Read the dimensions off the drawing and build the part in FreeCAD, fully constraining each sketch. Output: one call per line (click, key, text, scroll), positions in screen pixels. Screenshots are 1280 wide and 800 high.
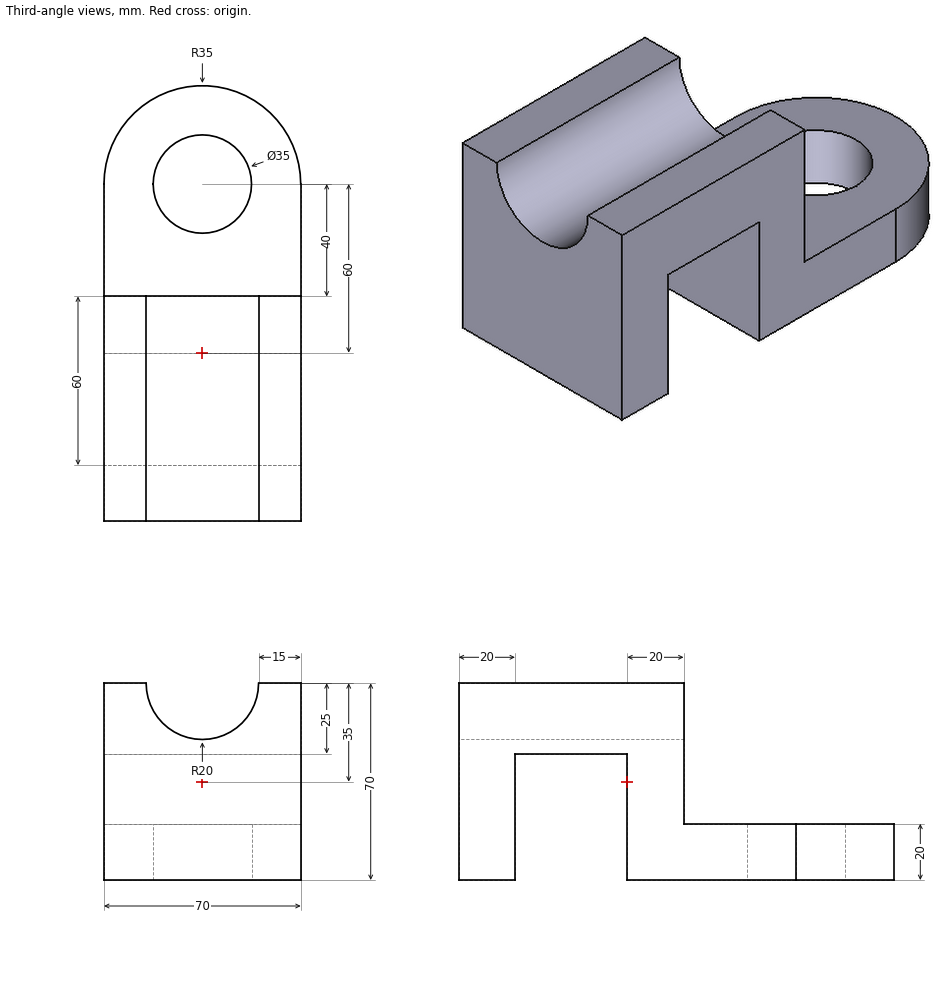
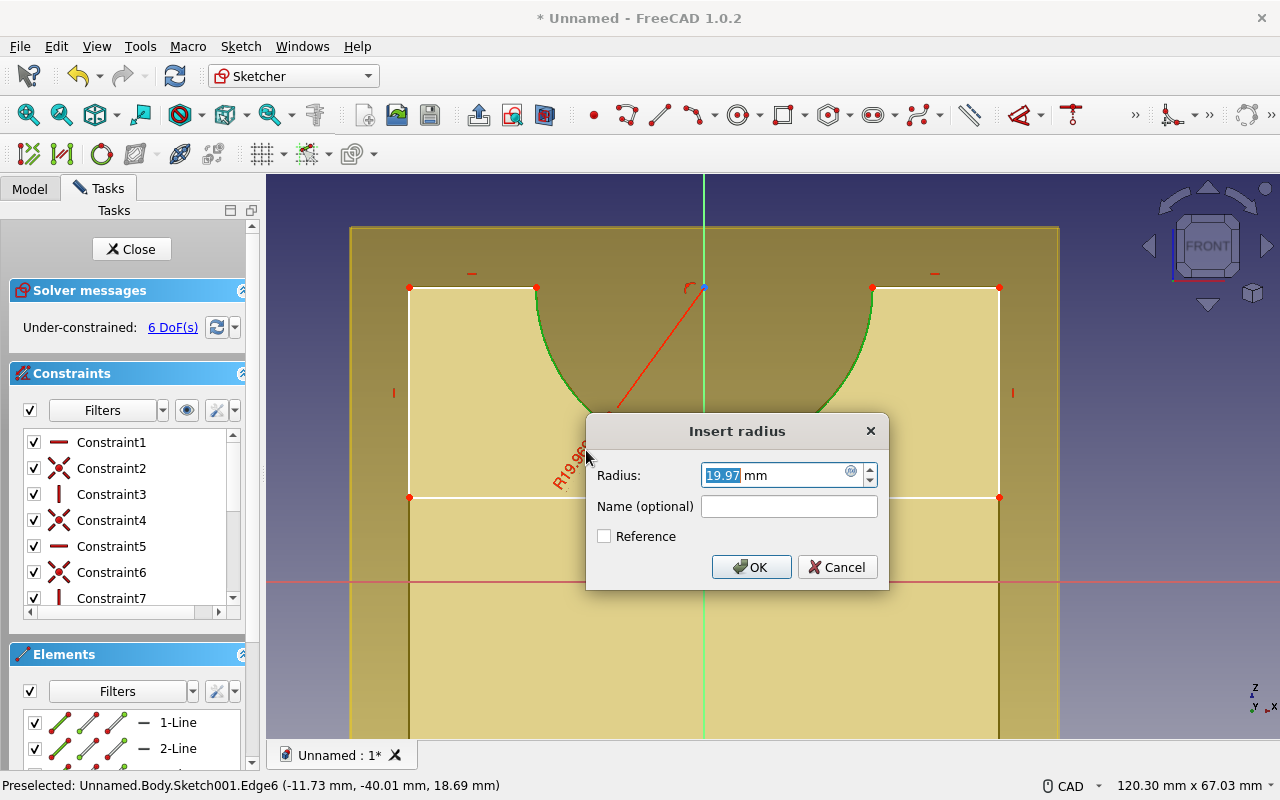
text(20)
key(Return)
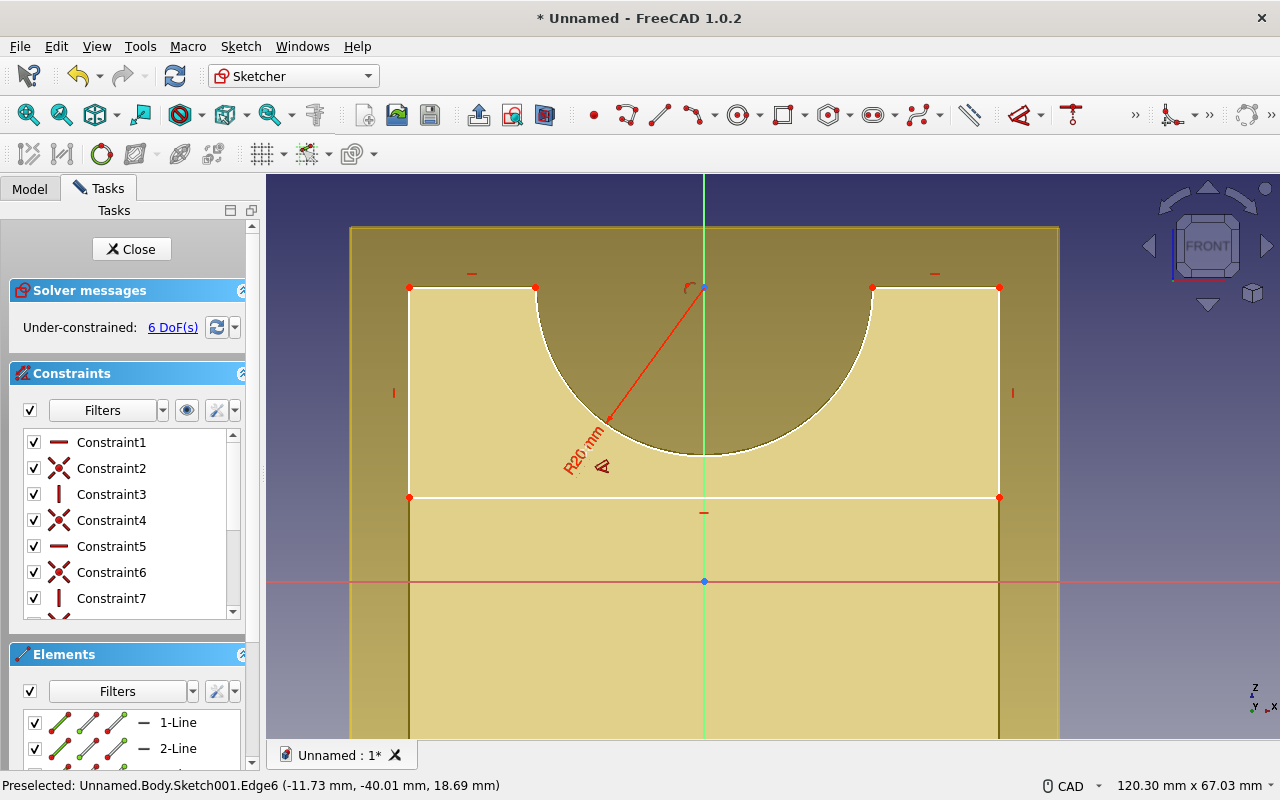
click(911, 288)
click(936, 254)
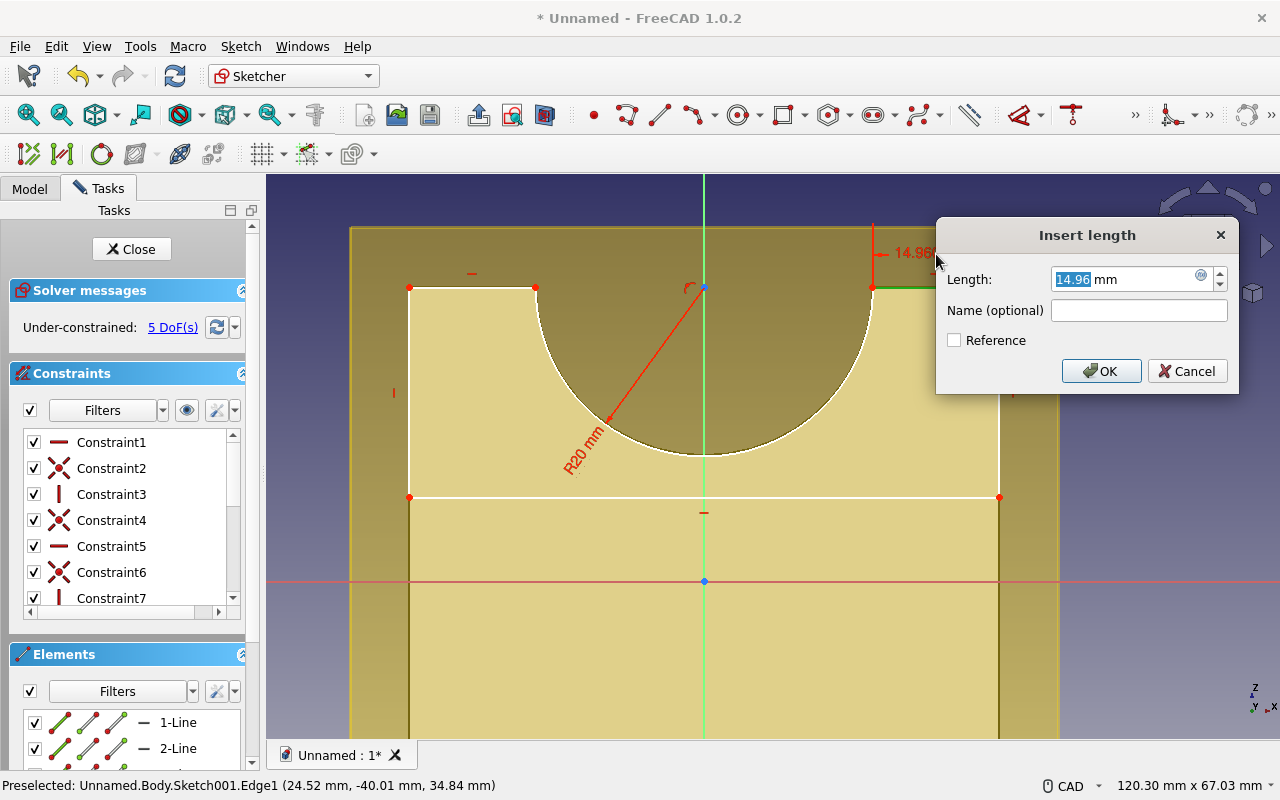
text(15)
key(Return)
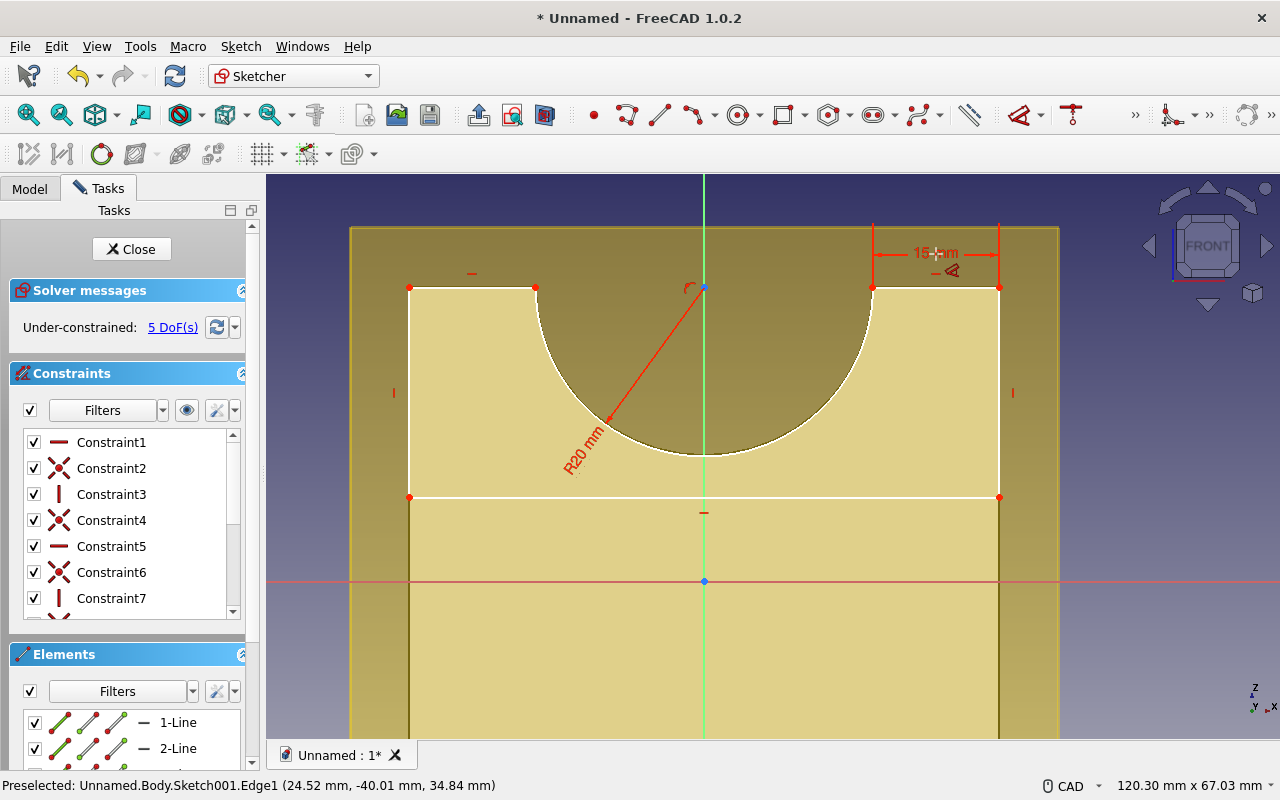
click(999, 351)
click(1033, 393)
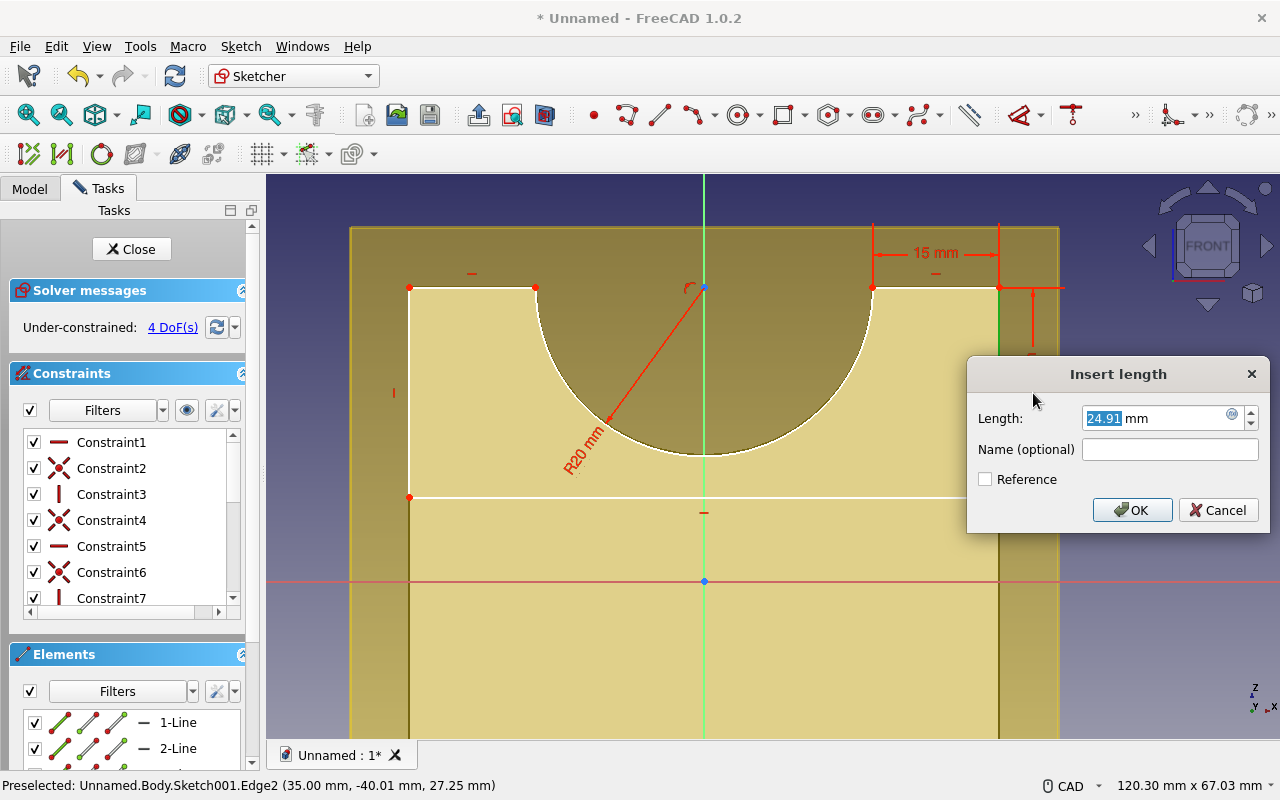
text(25)
key(Return)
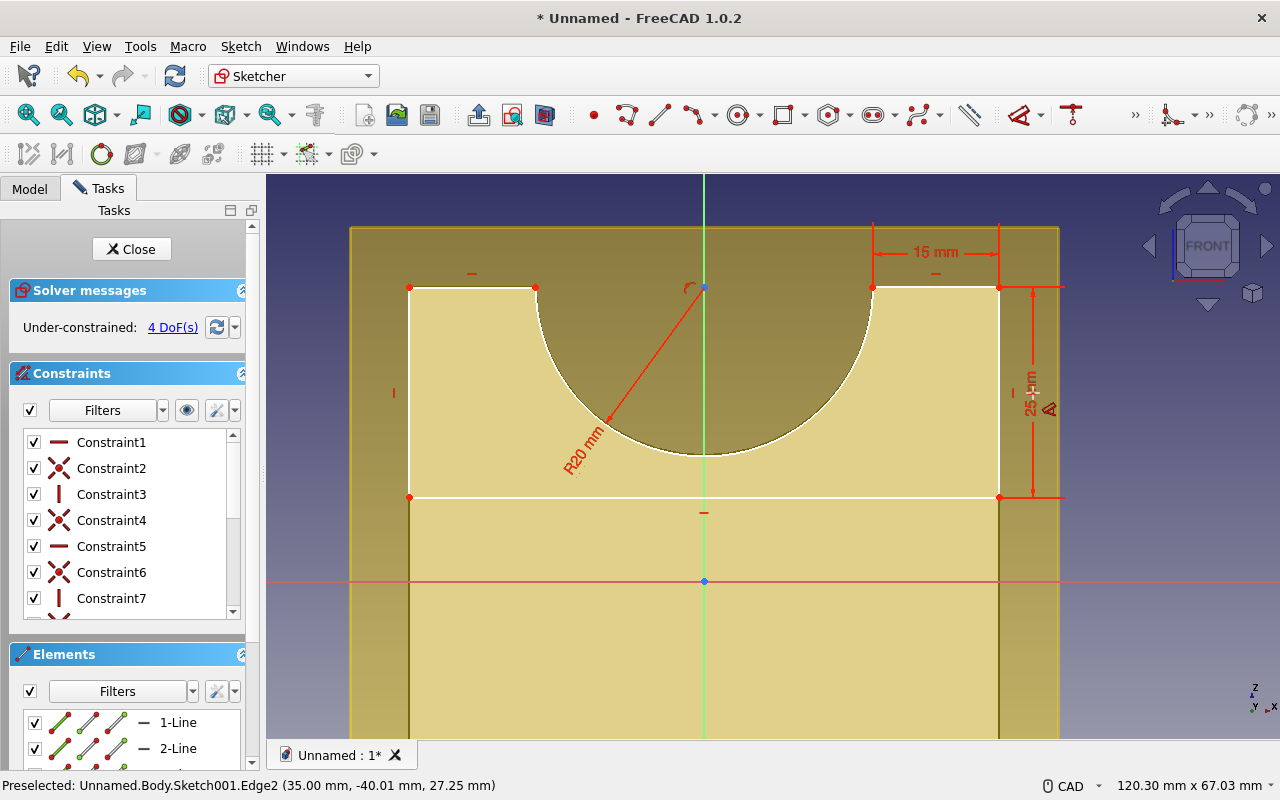
click(822, 498)
click(568, 532)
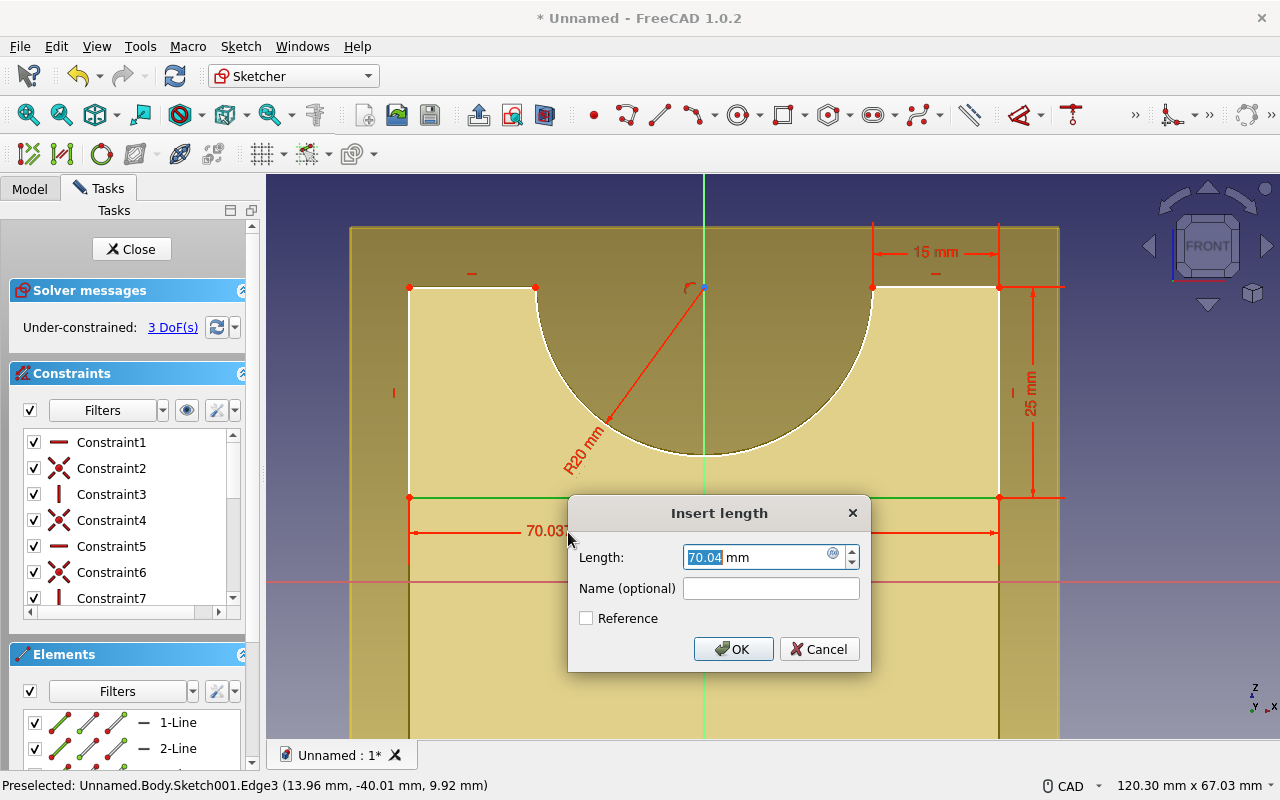
text(70)
key(Return)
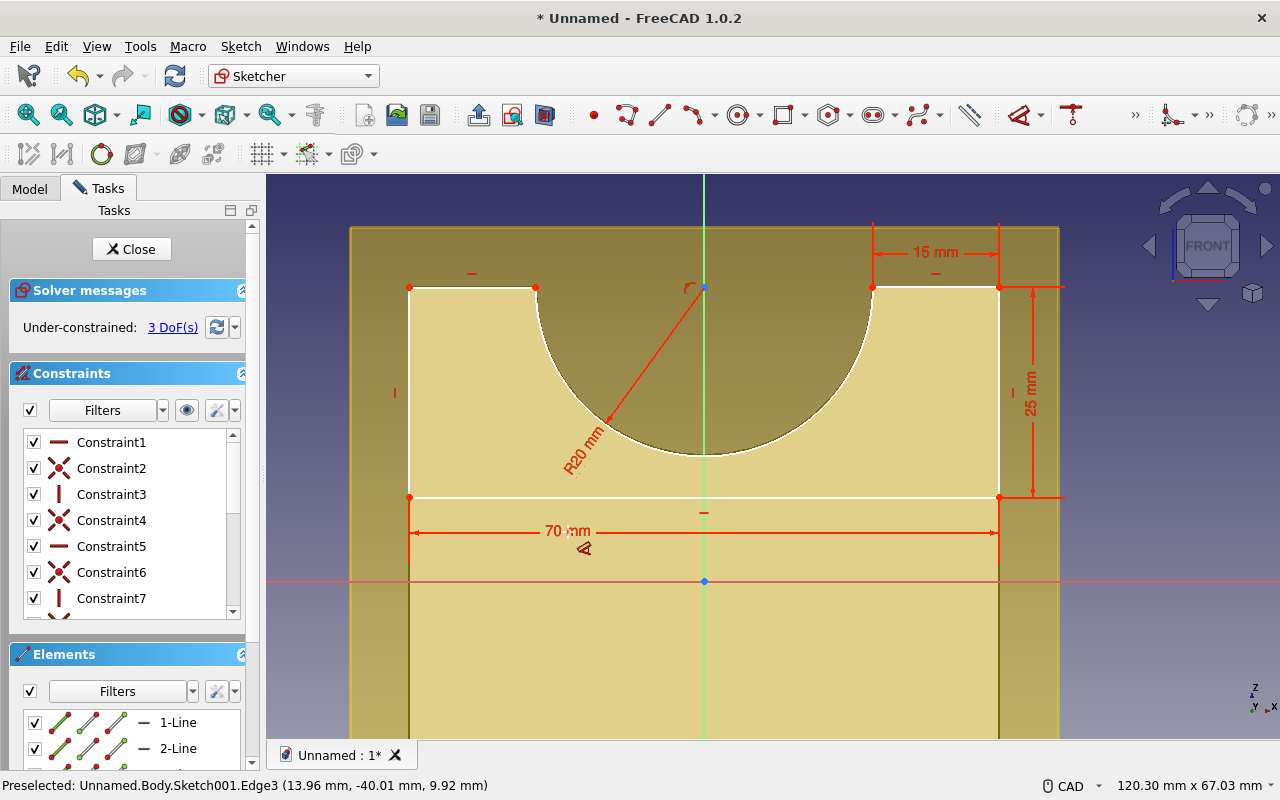
click(409, 435)
click(375, 393)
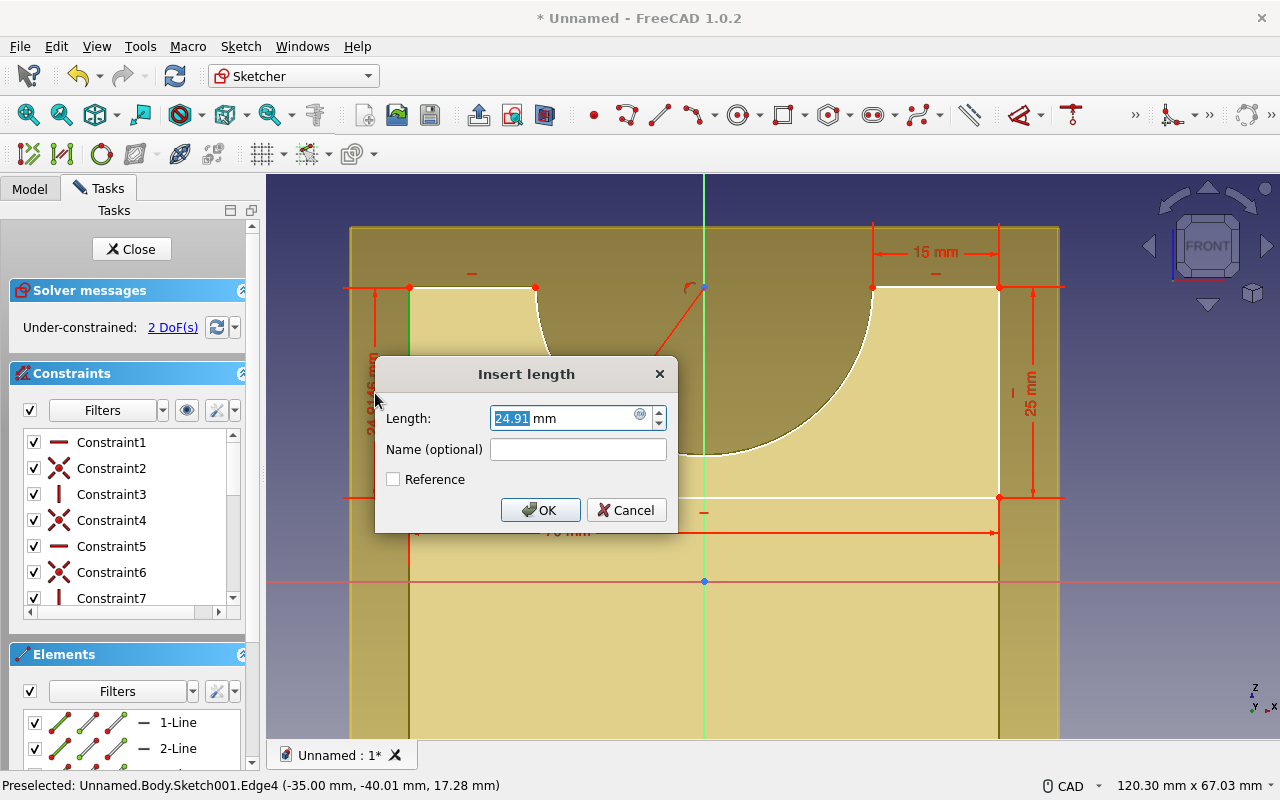
text(25)
key(Return)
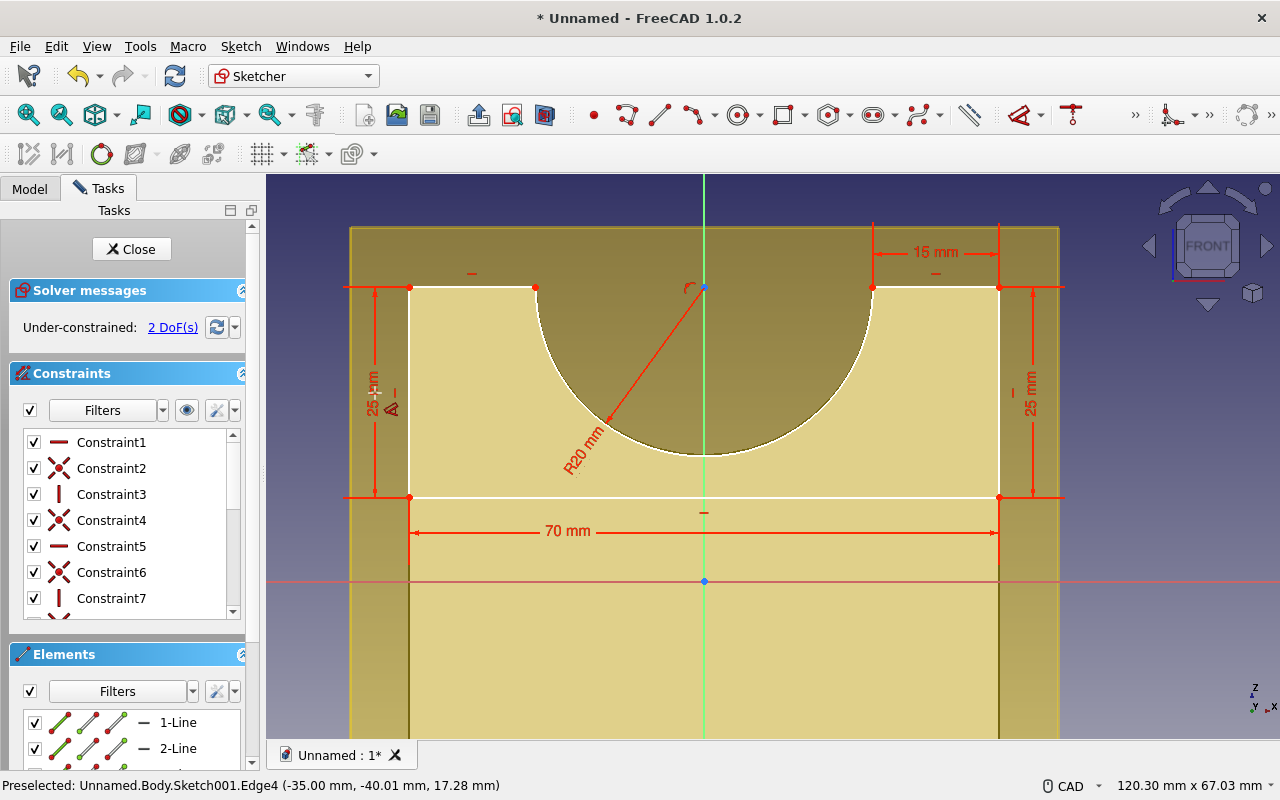
click(873, 287)
click(907, 434)